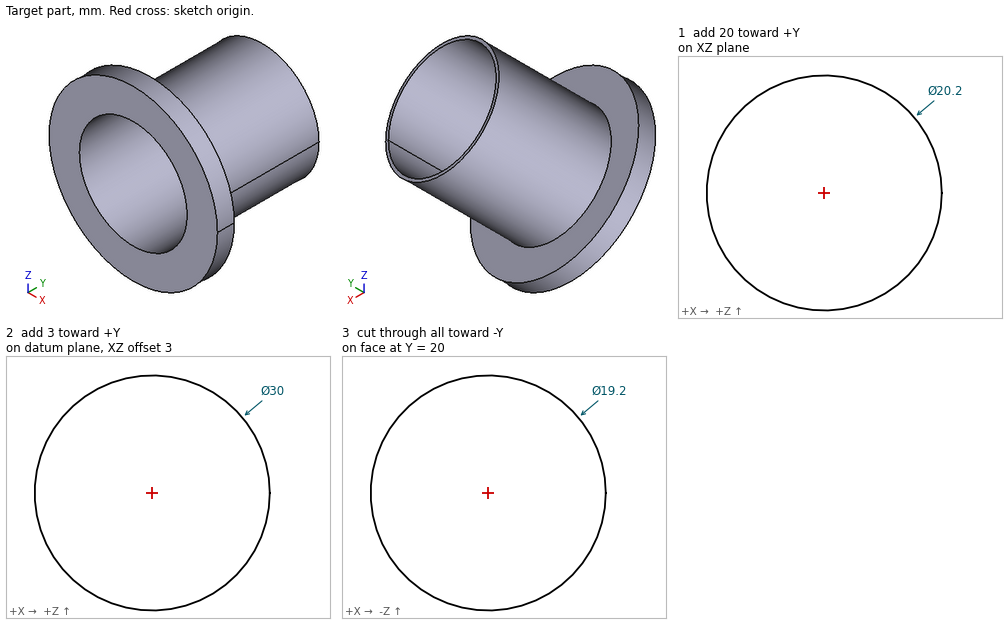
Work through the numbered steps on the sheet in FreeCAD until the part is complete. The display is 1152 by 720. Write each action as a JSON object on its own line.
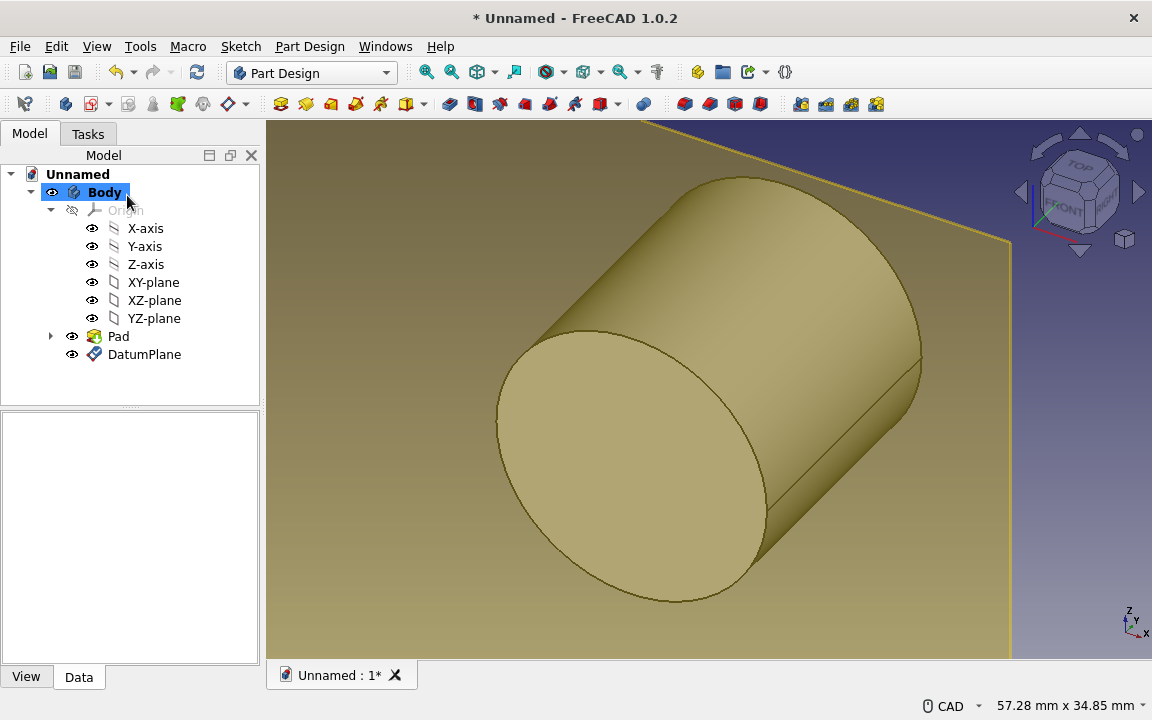
{"action": "left_click", "coordinate": [117, 354]}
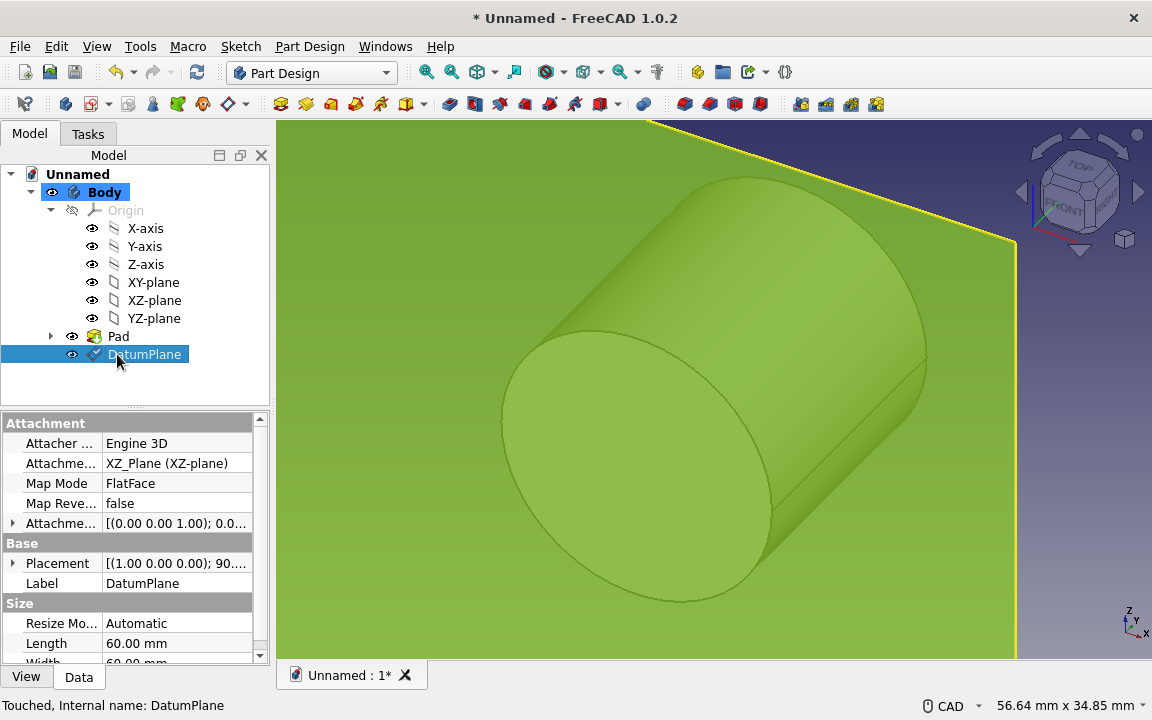
{"action": "left_click", "coordinate": [90, 104]}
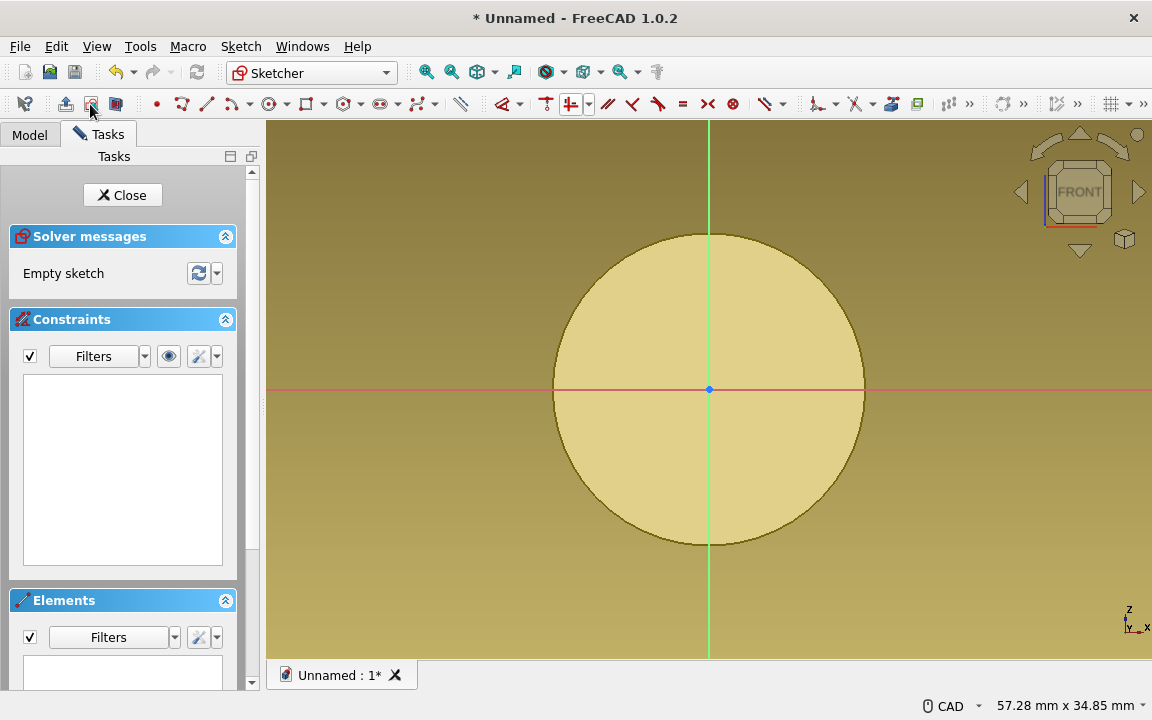
{"action": "scroll", "coordinate": [501, 389], "scroll_direction": "down", "scroll_amount": 2}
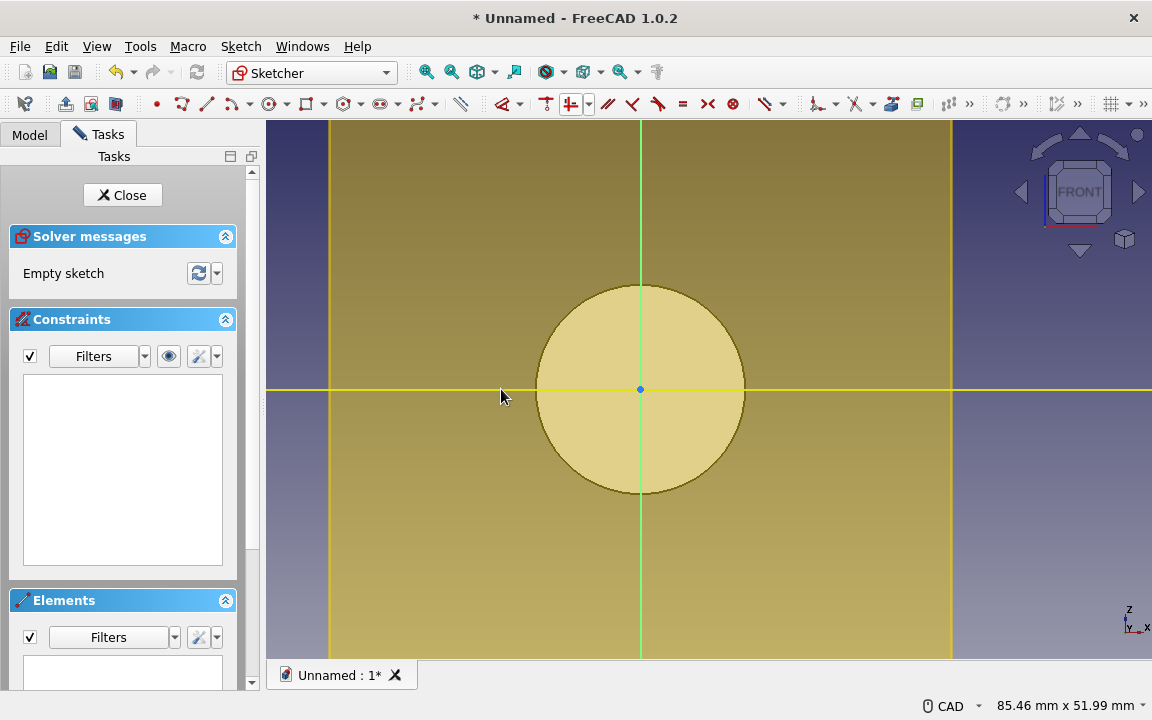
{"action": "key", "text": "g c"}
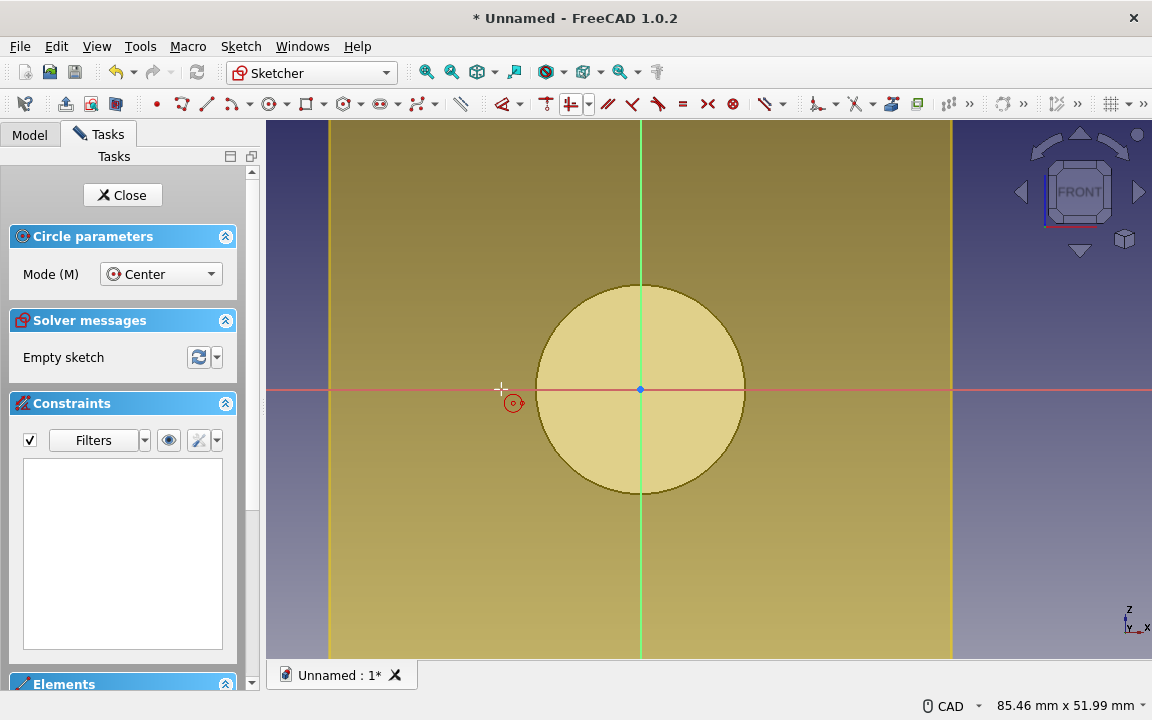
{"action": "left_click", "coordinate": [641, 390]}
{"action": "left_click", "coordinate": [750, 280]}
{"action": "key", "text": "Escape"}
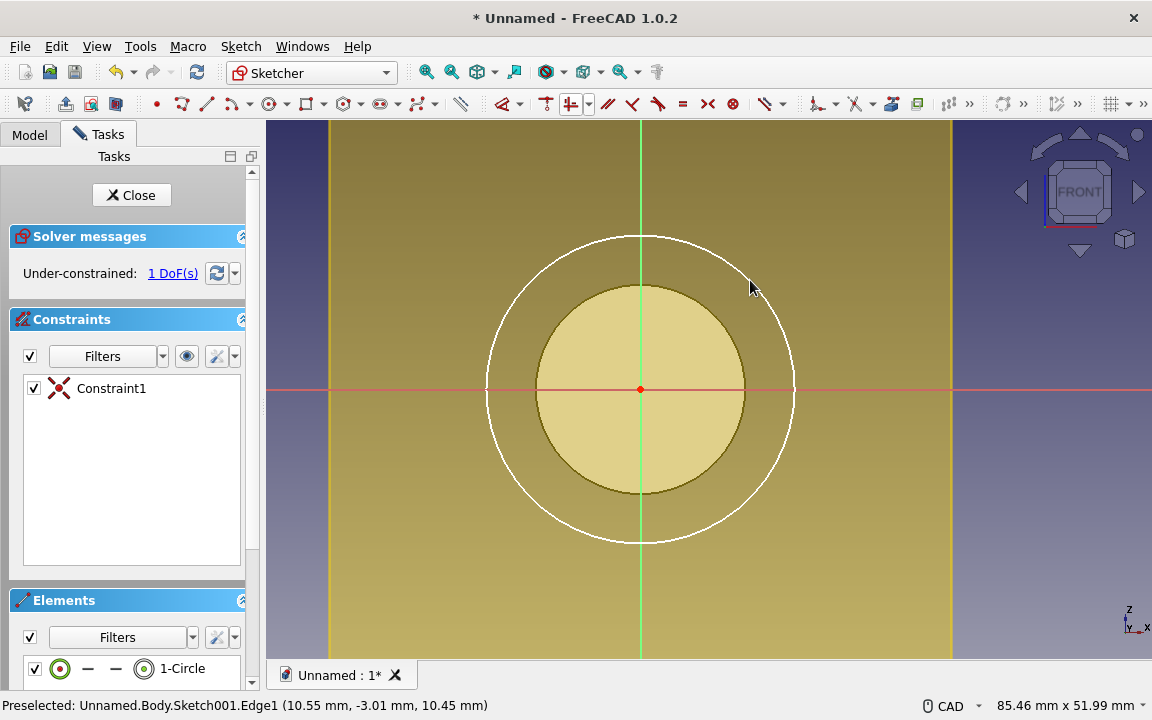
{"action": "left_click", "coordinate": [502, 104]}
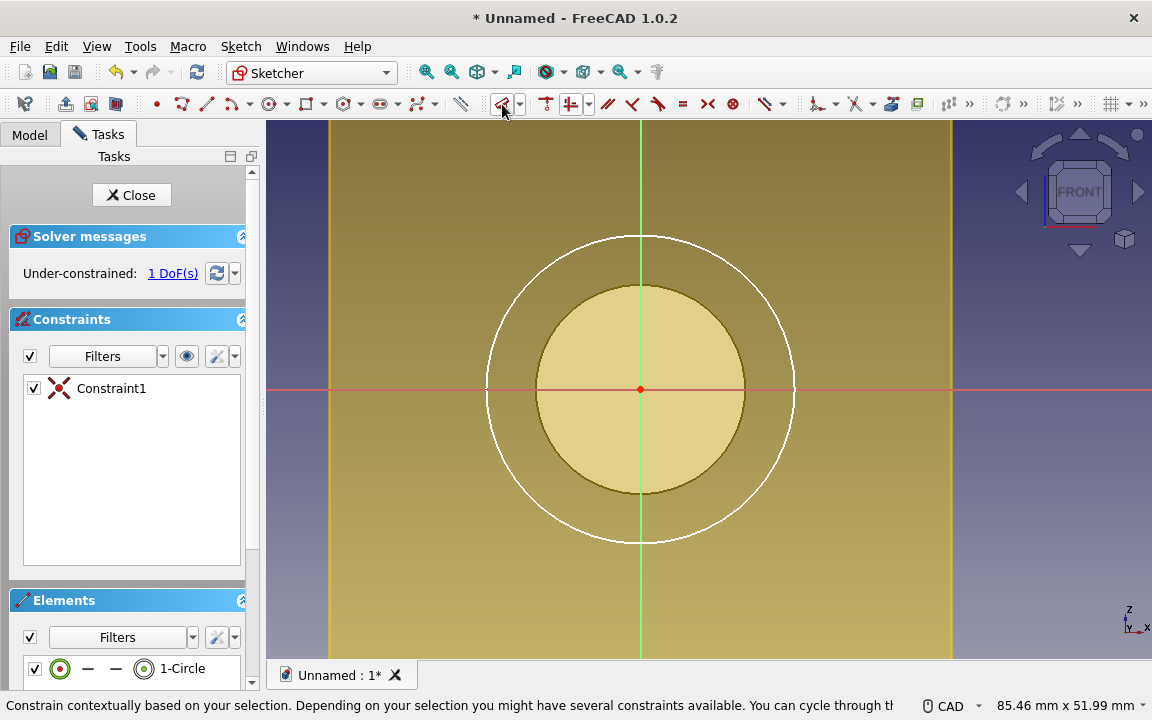
{"action": "left_click", "coordinate": [749, 280]}
{"action": "left_click", "coordinate": [772, 257]}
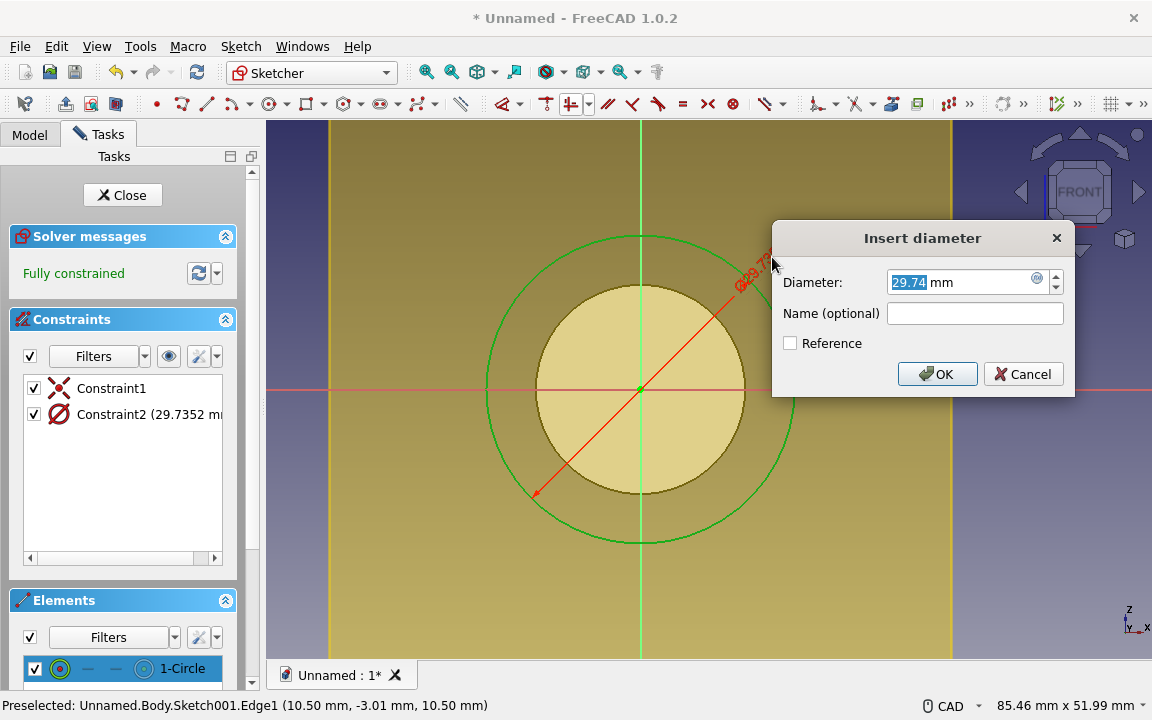
{"action": "type", "text": "30"}
{"action": "key", "text": "Return"}
{"action": "key", "text": "Escape"}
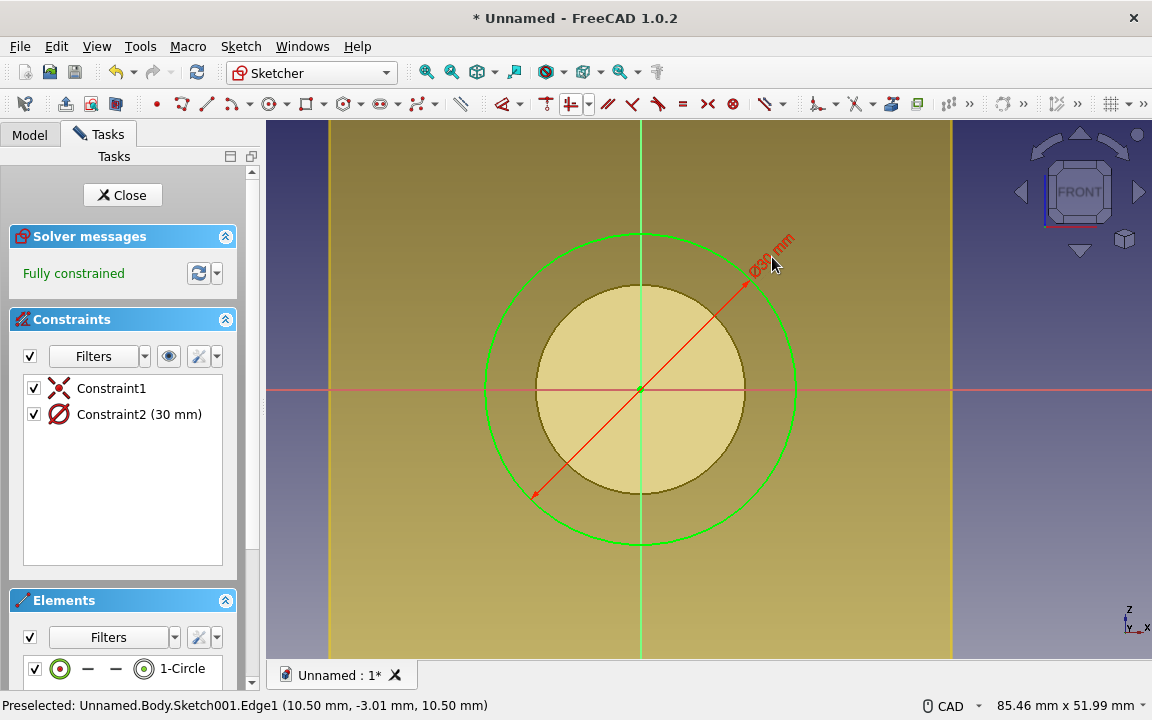
{"action": "left_click", "coordinate": [123, 195]}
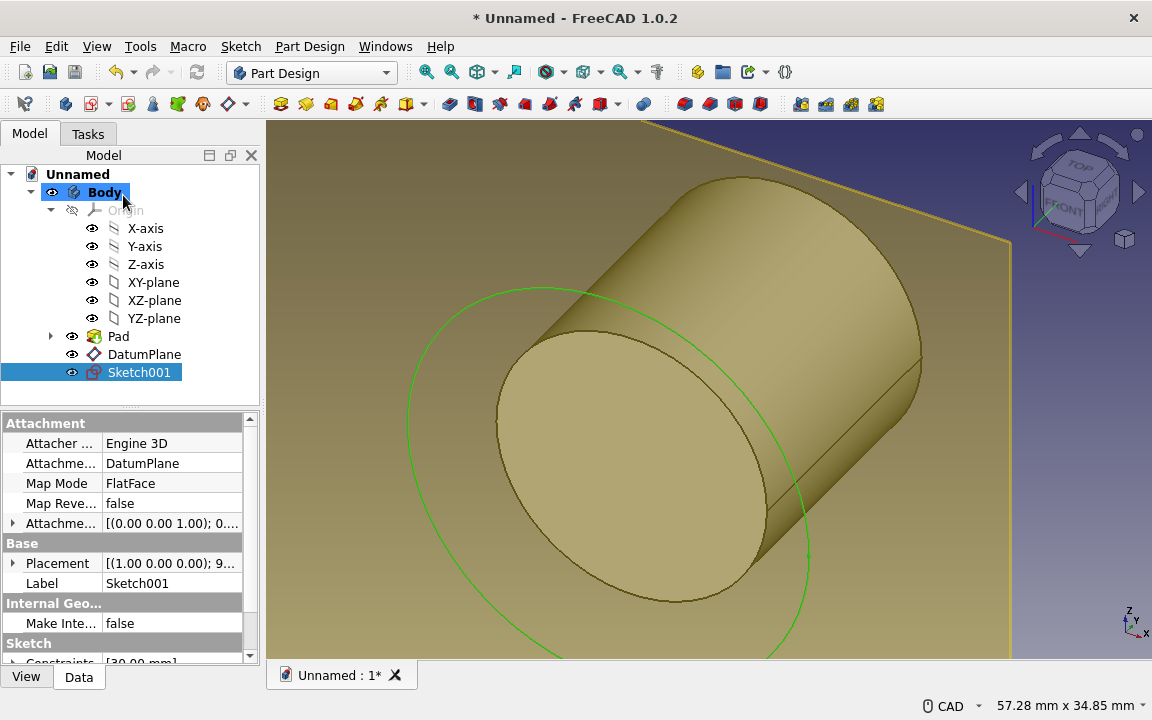
{"action": "left_click", "coordinate": [281, 104]}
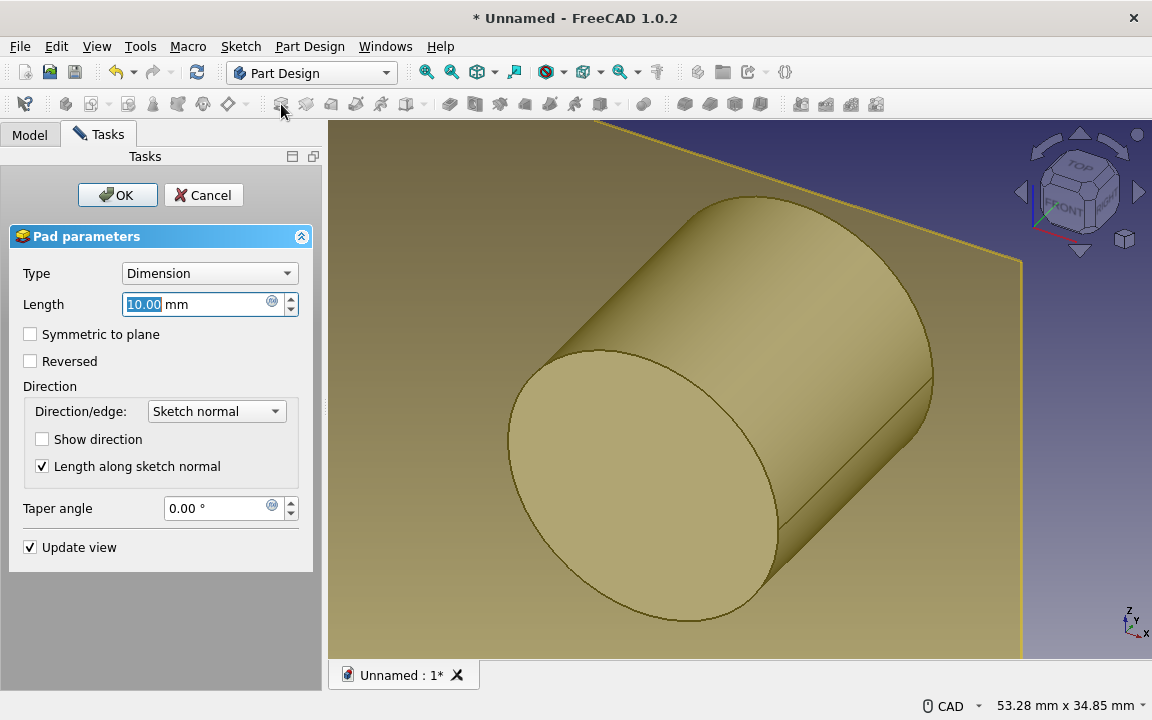
{"action": "type", "text": "3"}
{"action": "key", "text": "Tab"}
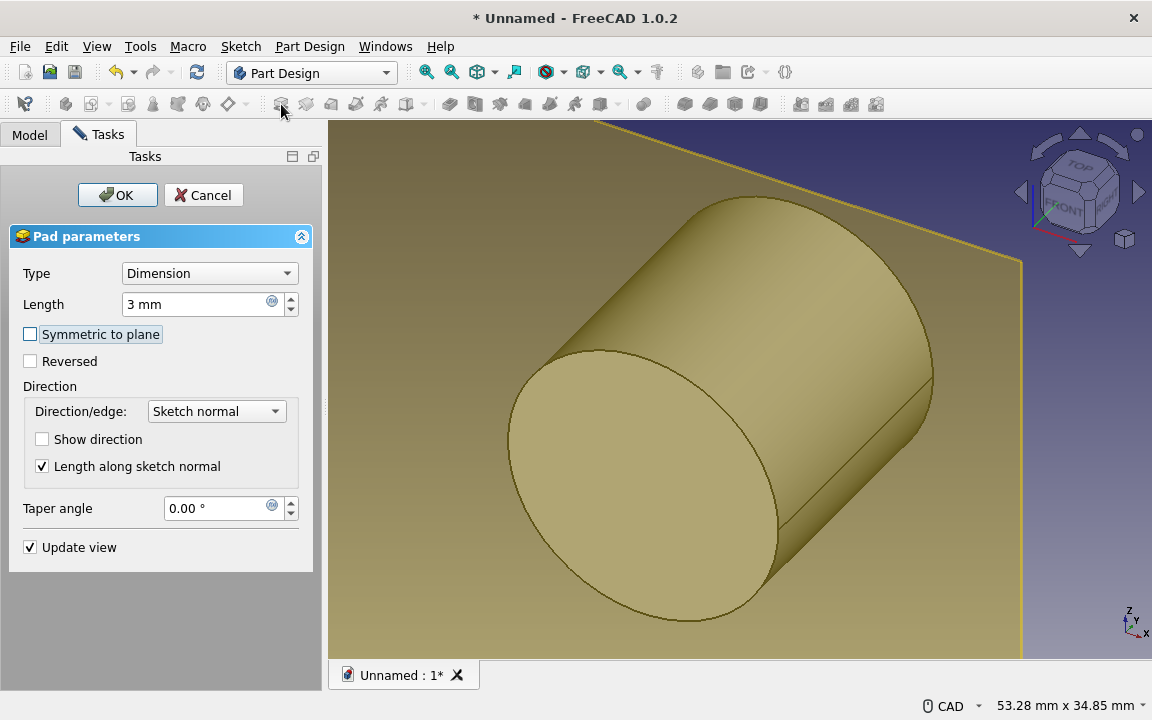
{"action": "left_click", "coordinate": [31, 361]}